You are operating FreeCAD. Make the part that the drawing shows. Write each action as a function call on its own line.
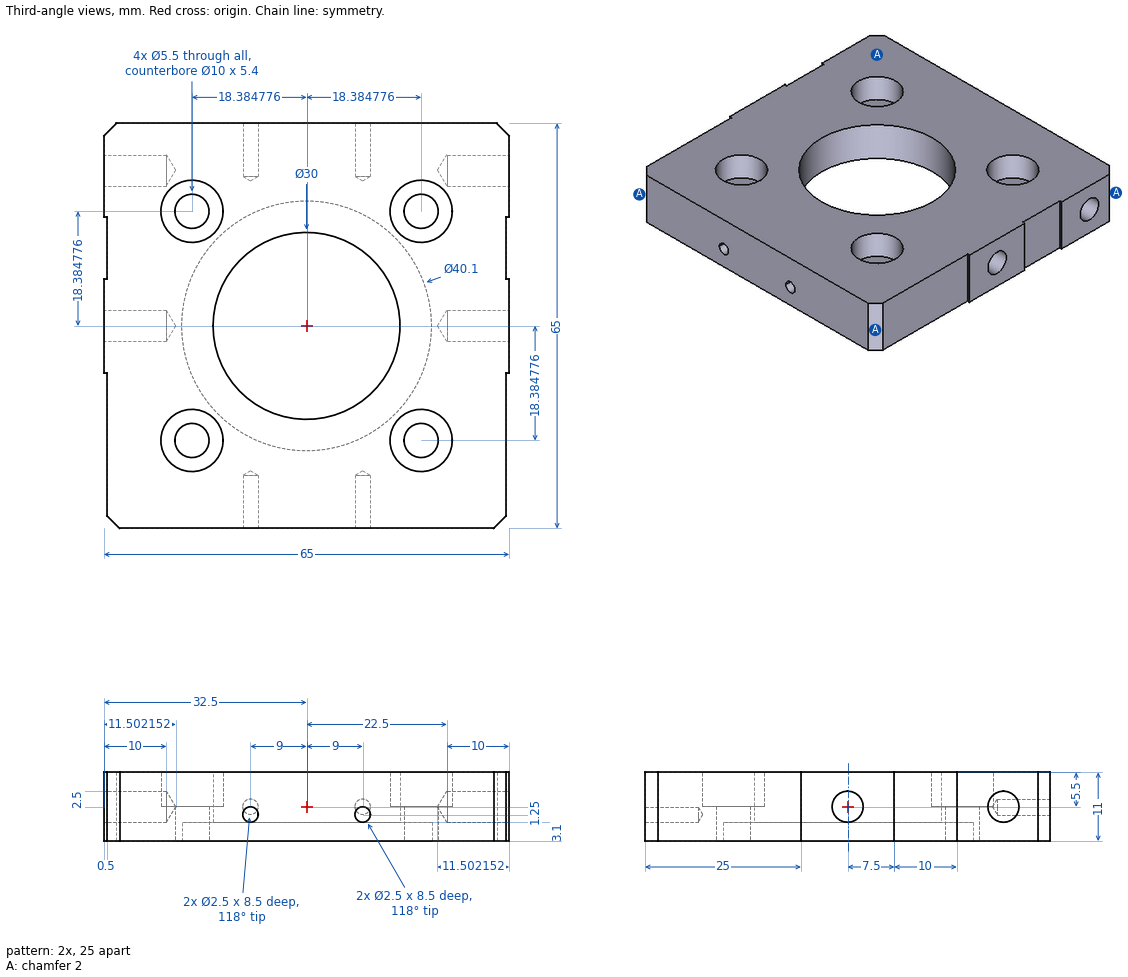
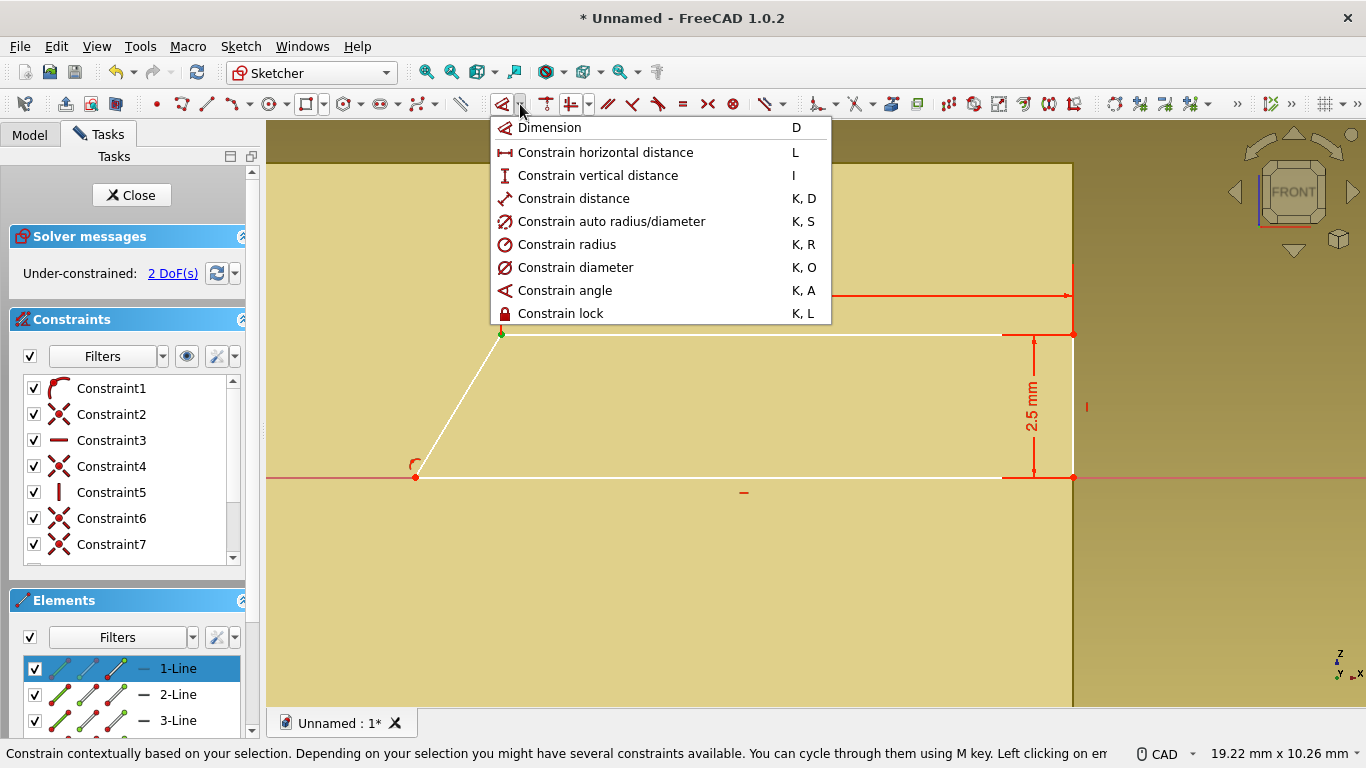
click(661, 152)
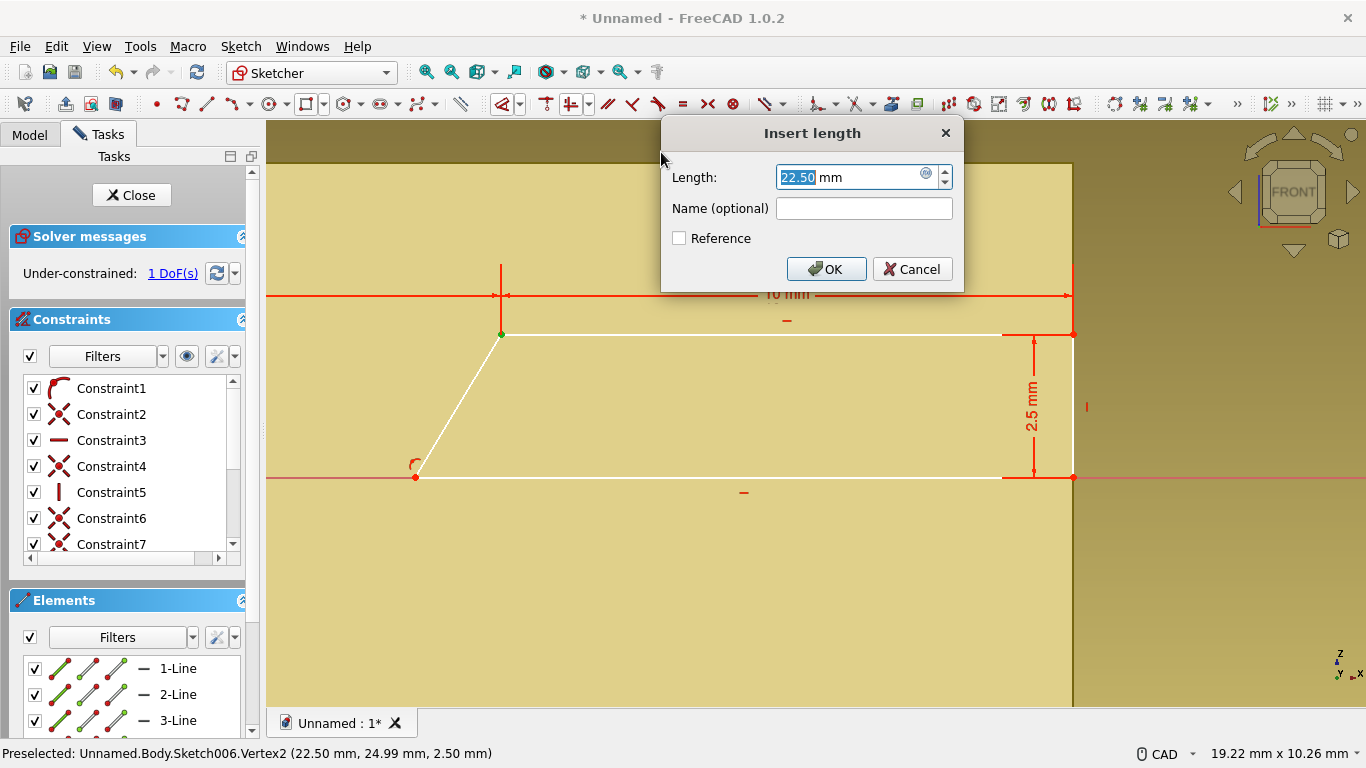
text(22.5)
key(Return)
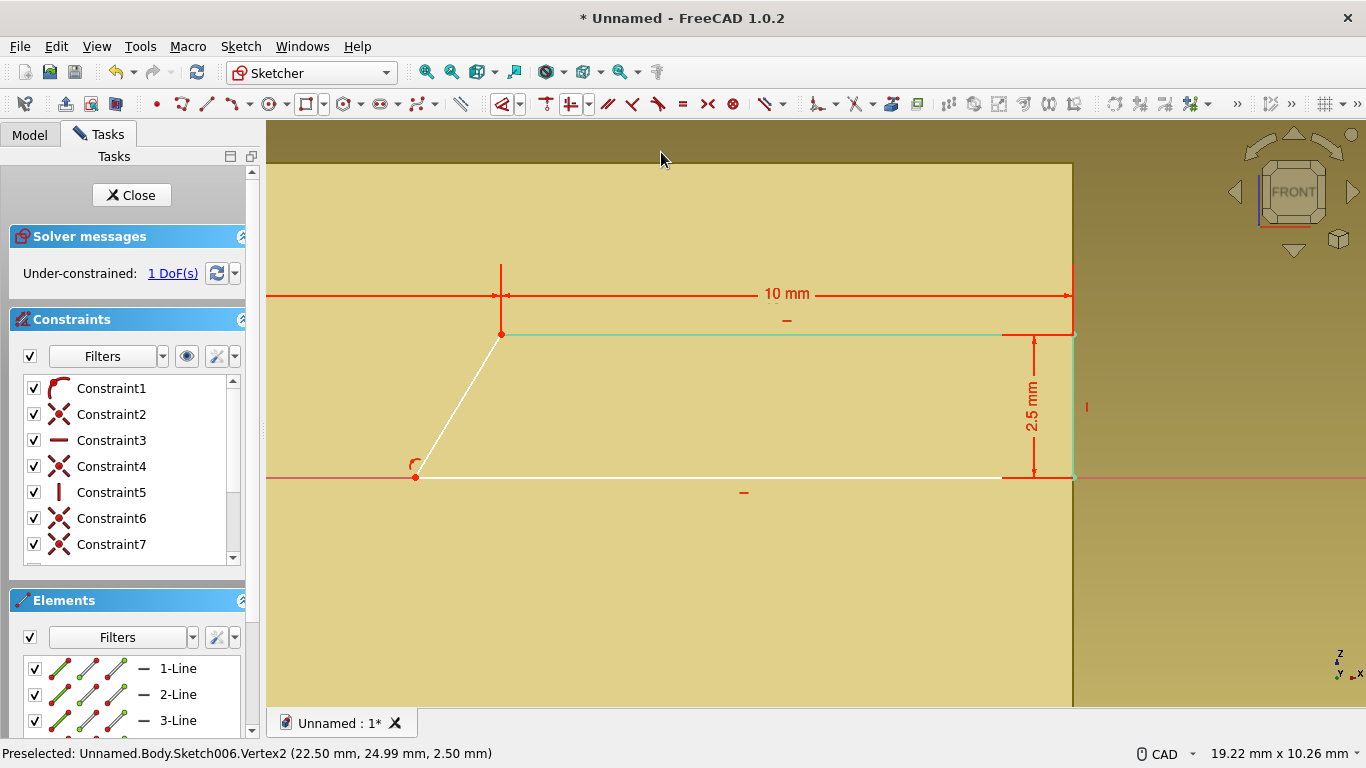
click(876, 478)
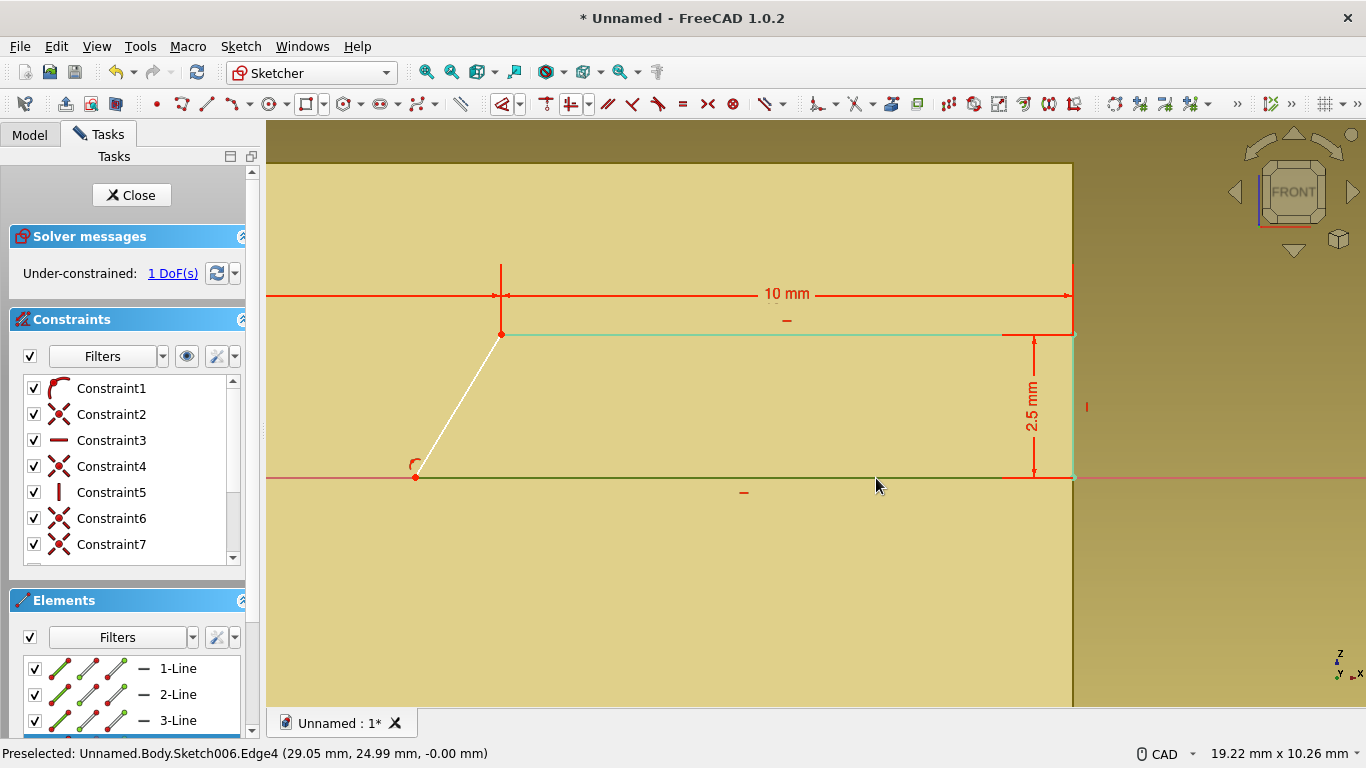
click(520, 104)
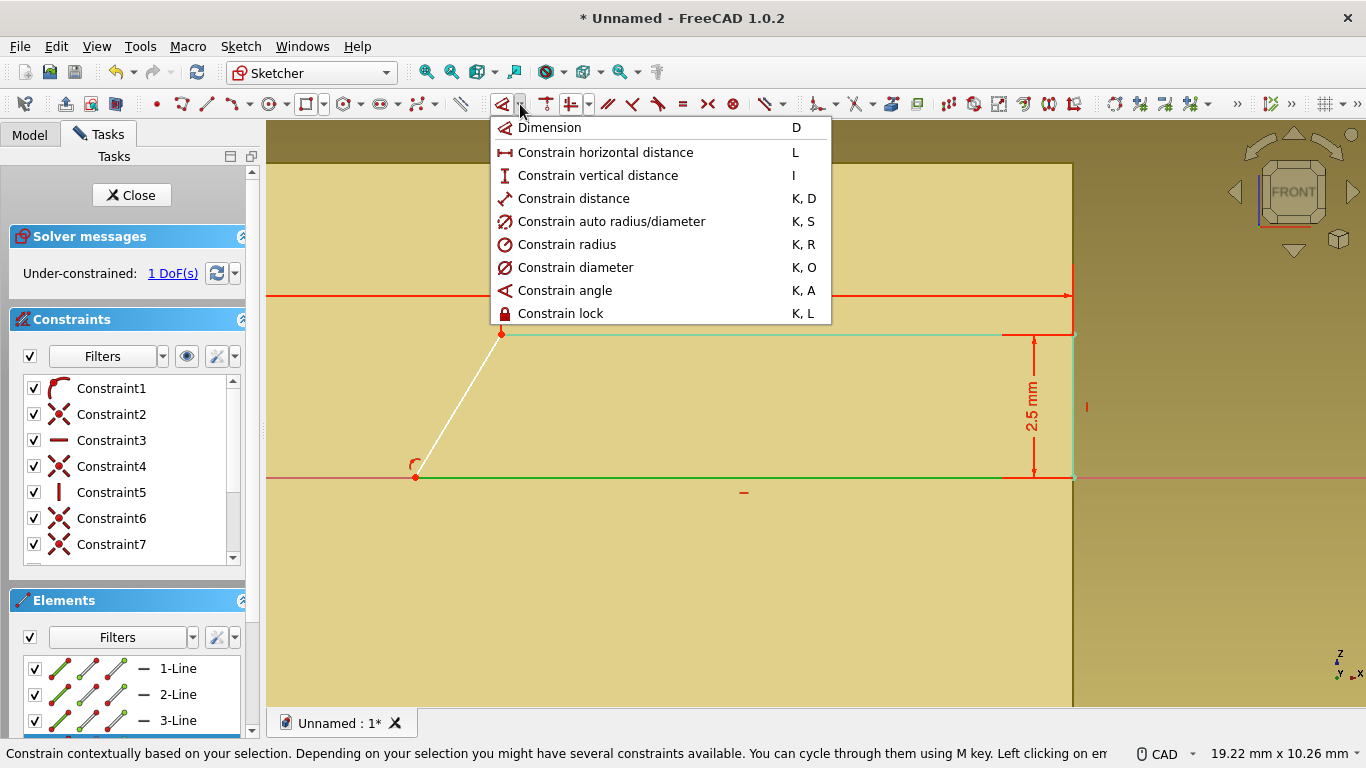
click(661, 152)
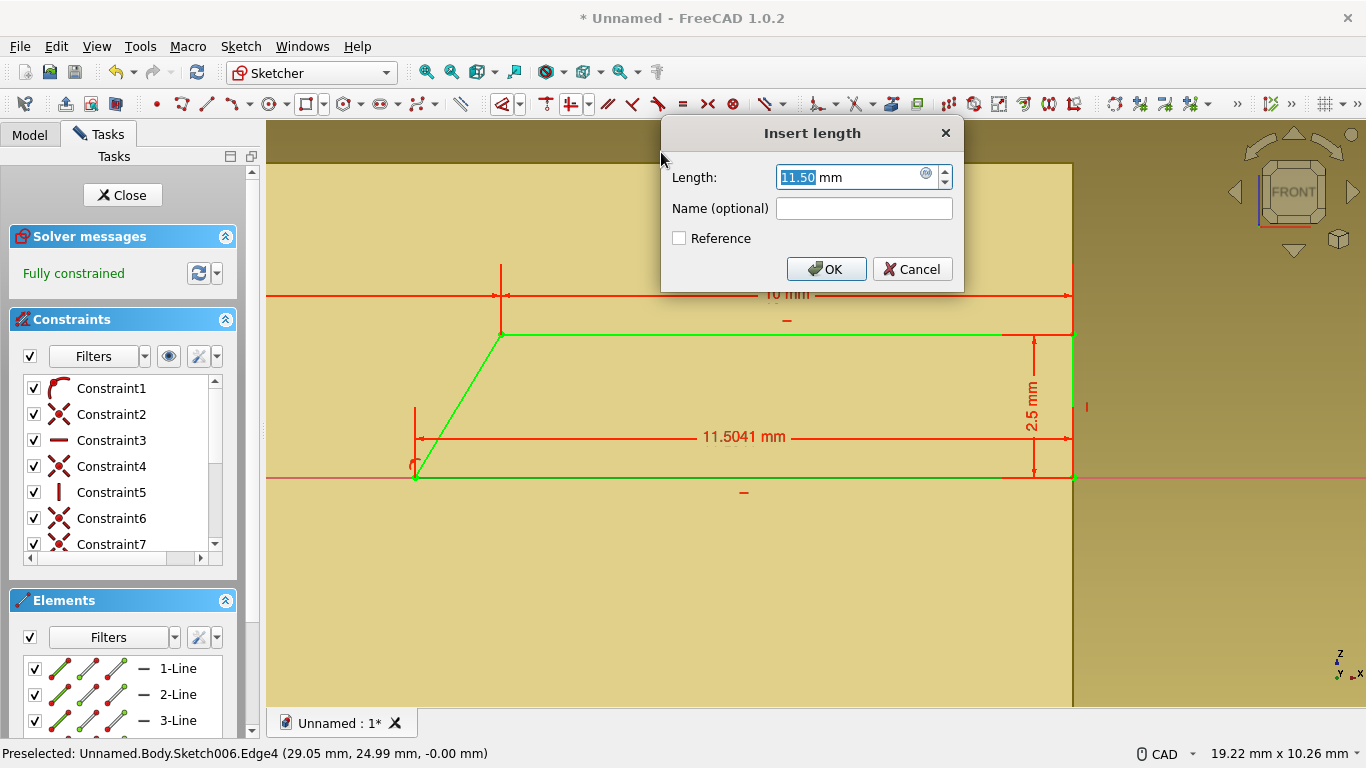
text(11.502152)
key(Return)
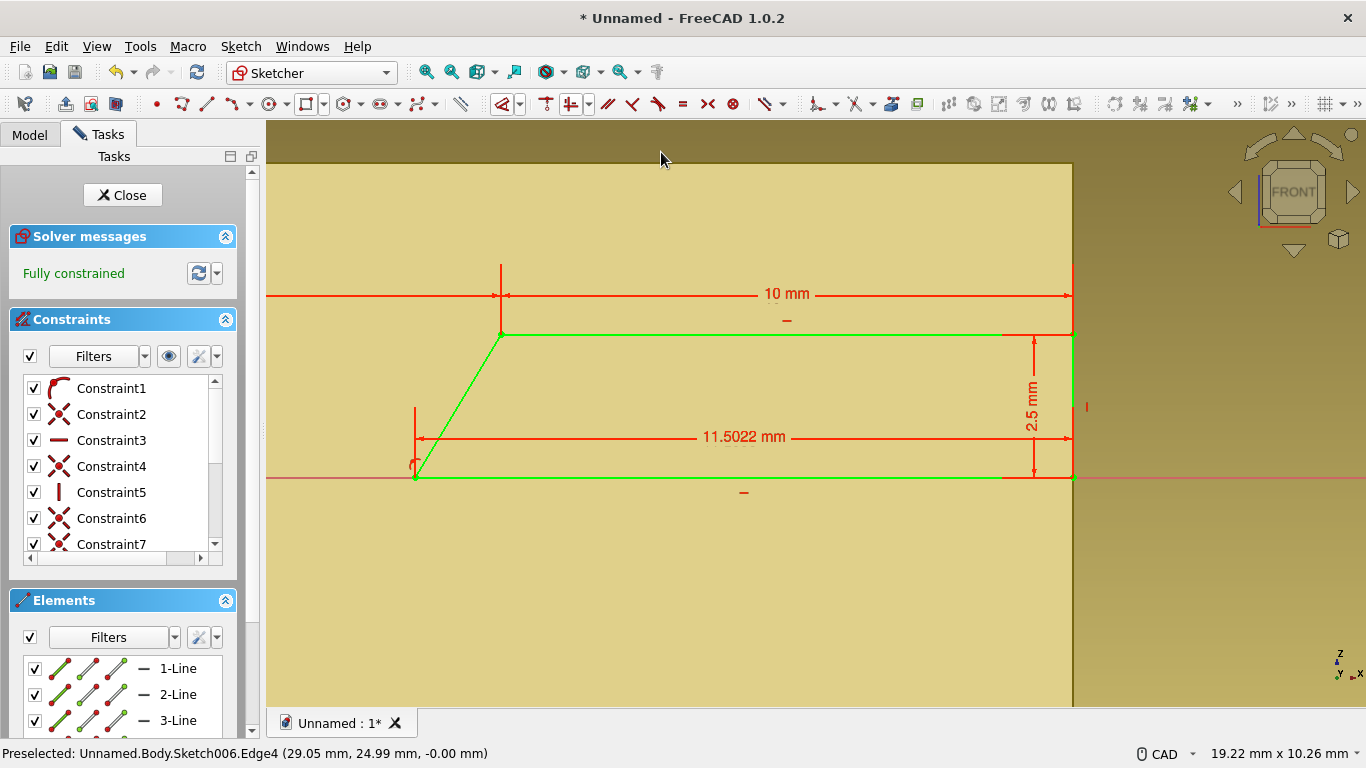
click(123, 195)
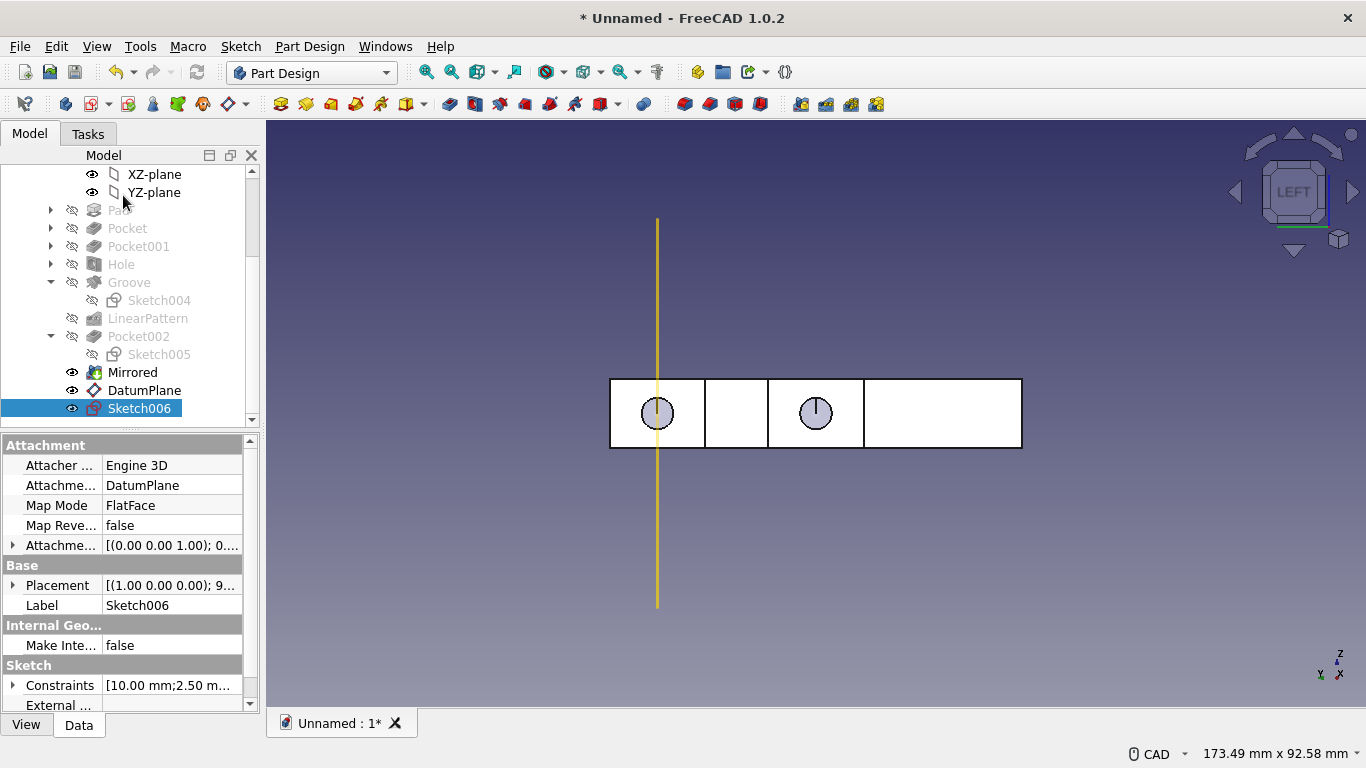
click(500, 104)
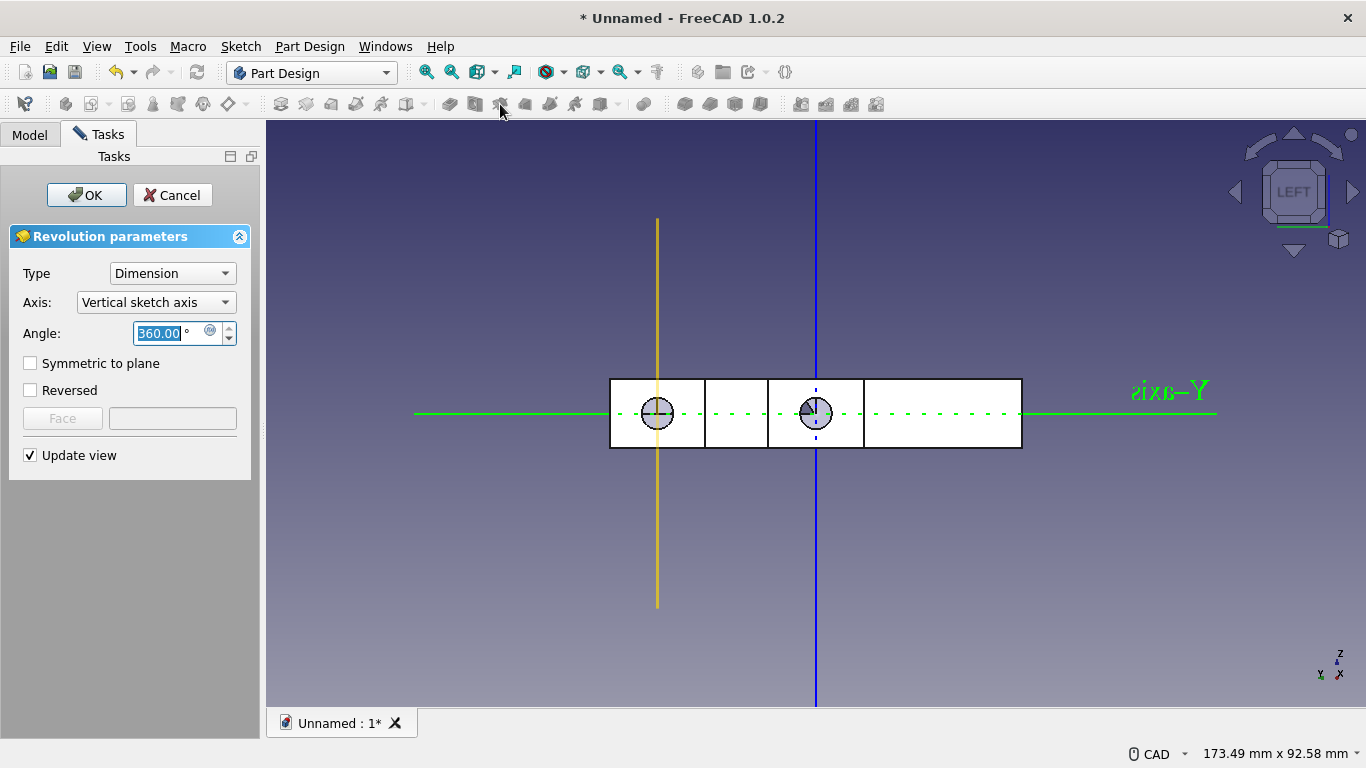
click(157, 302)